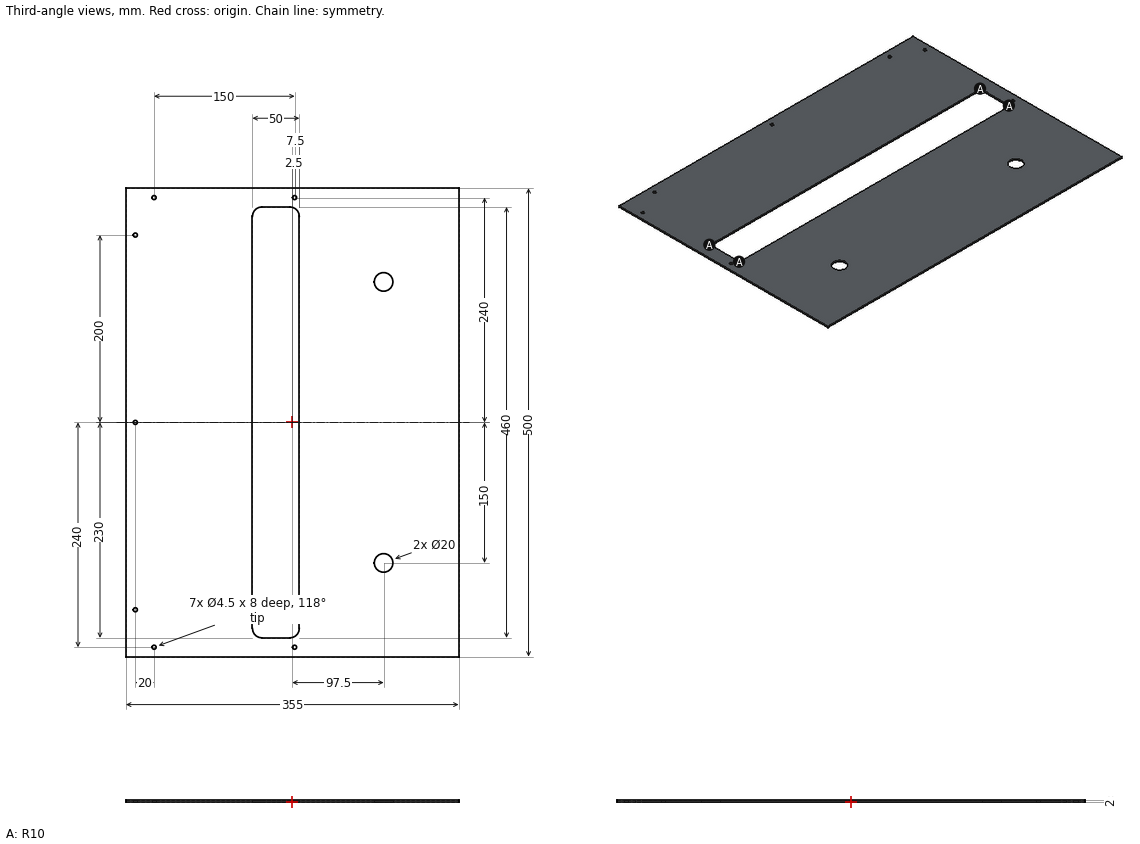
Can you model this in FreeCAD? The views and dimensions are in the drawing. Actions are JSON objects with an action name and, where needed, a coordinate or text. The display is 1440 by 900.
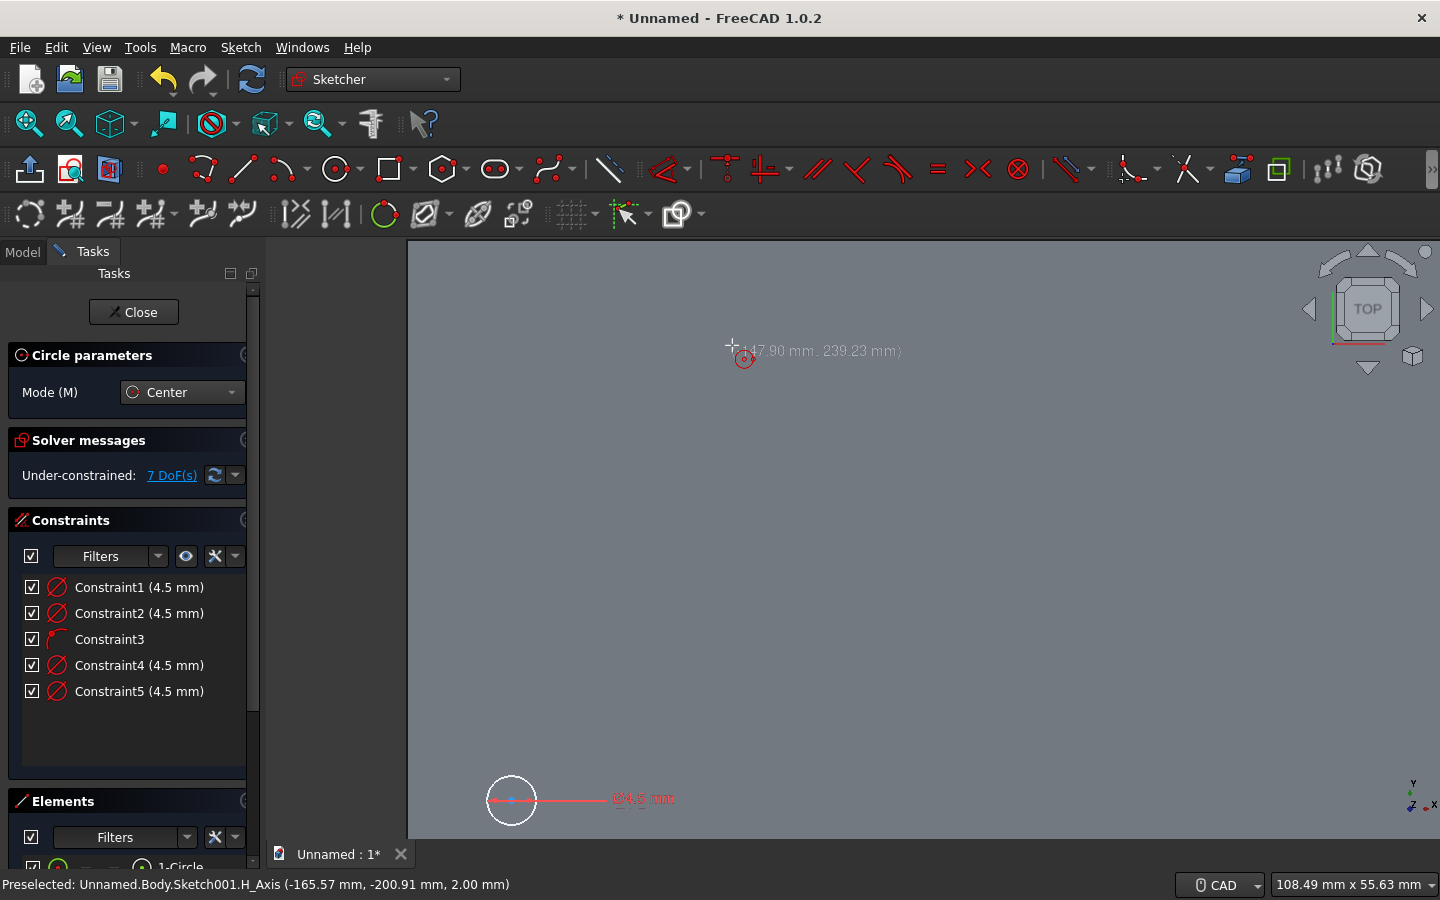
{"action": "scroll", "coordinate": [732, 345], "scroll_direction": "down", "scroll_amount": 13}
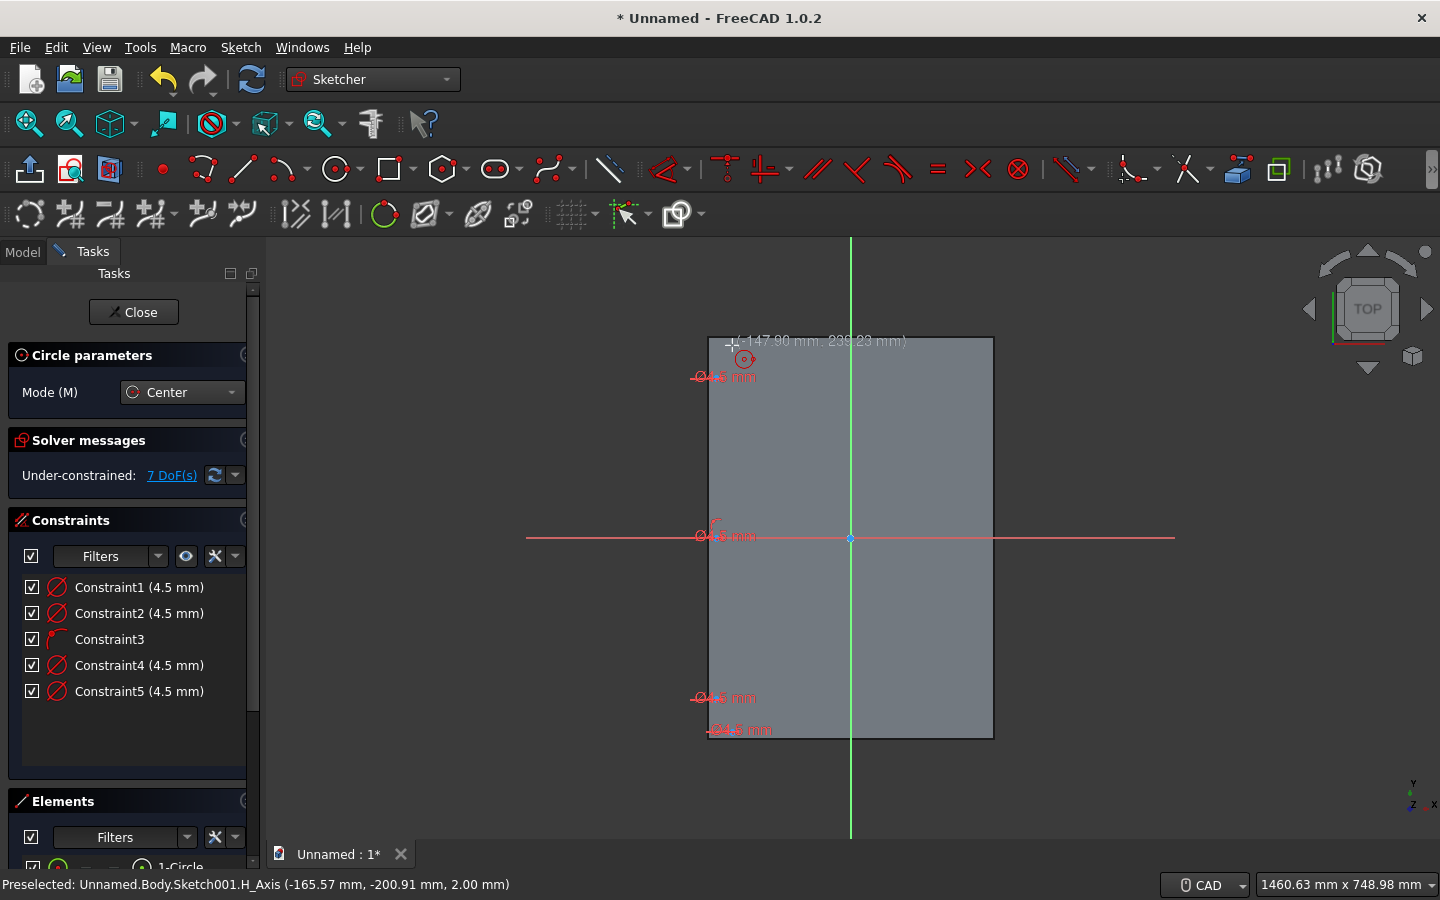
{"action": "left_click", "coordinate": [732, 345]}
{"action": "mouse_move", "coordinate": [734, 344]}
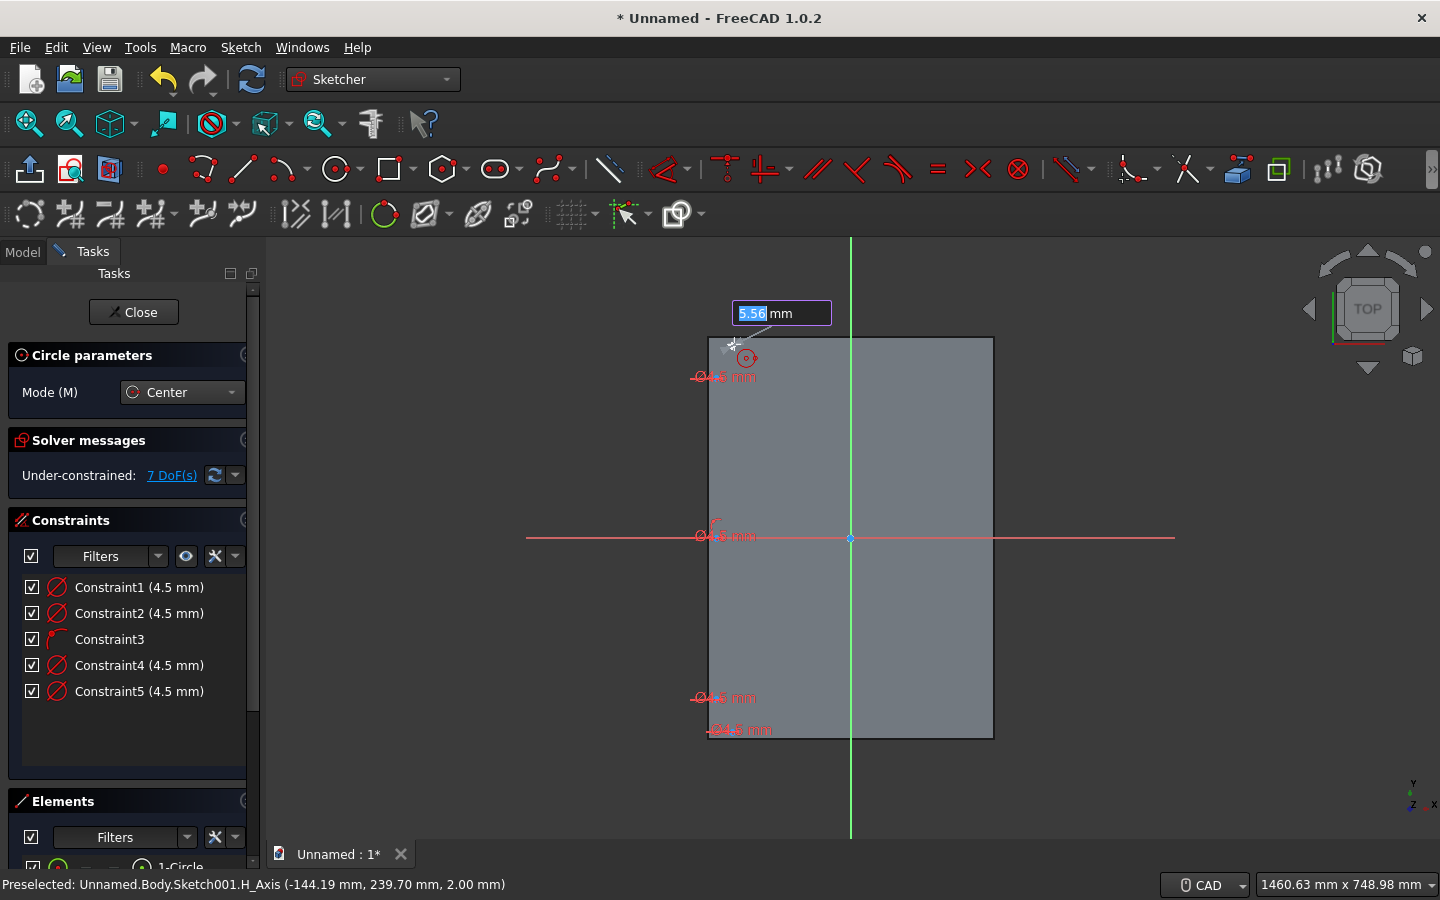
{"action": "type", "text": "4.5"}
{"action": "key", "text": "Return"}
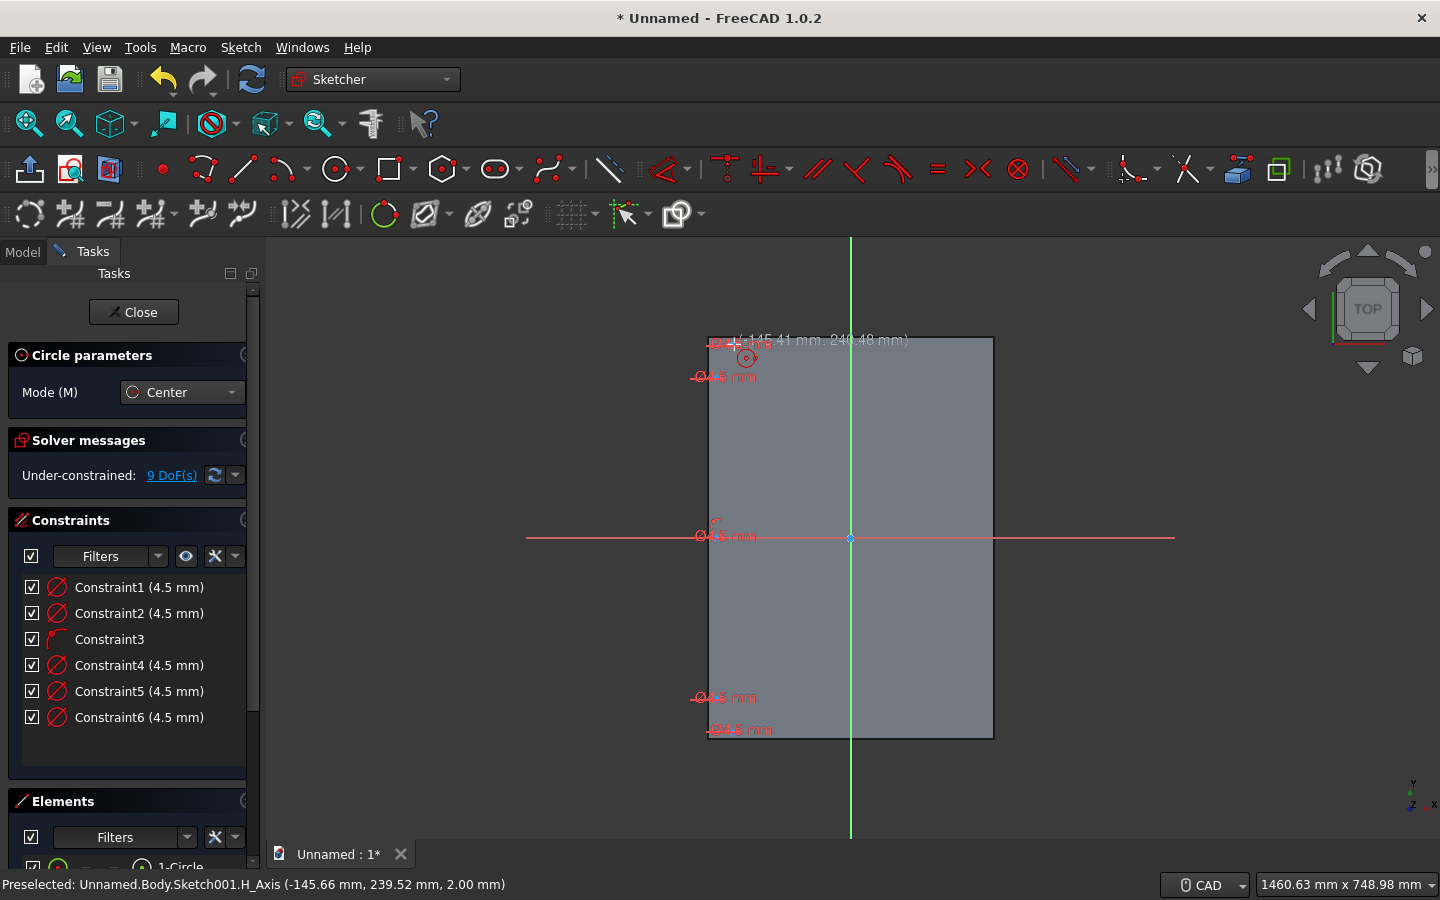
{"action": "scroll", "coordinate": [853, 345], "scroll_direction": "up", "scroll_amount": 13}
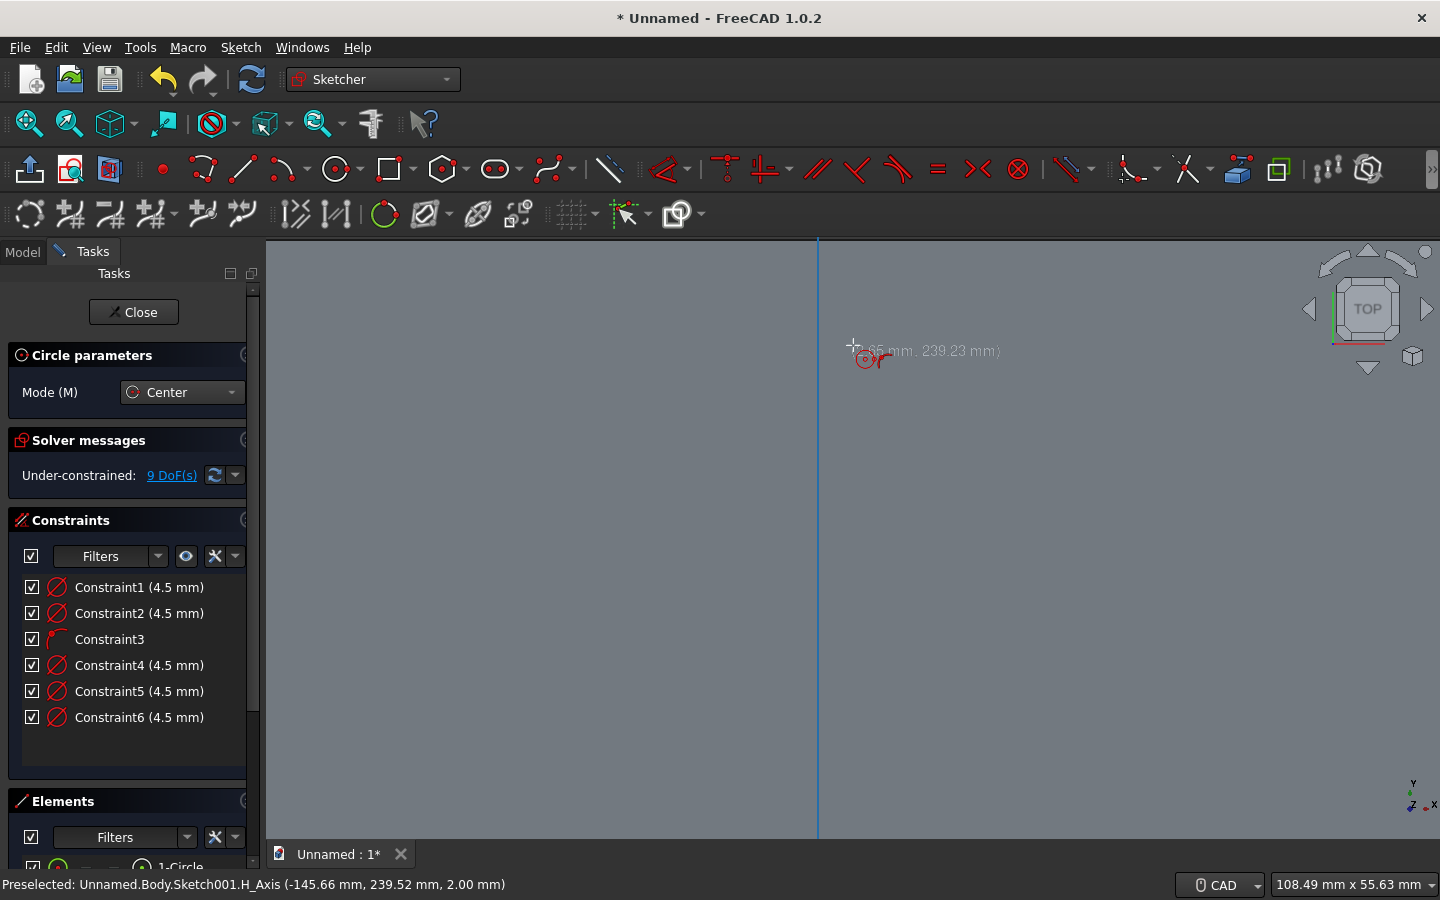
{"action": "left_click", "coordinate": [845, 348]}
{"action": "mouse_move", "coordinate": [862, 331]}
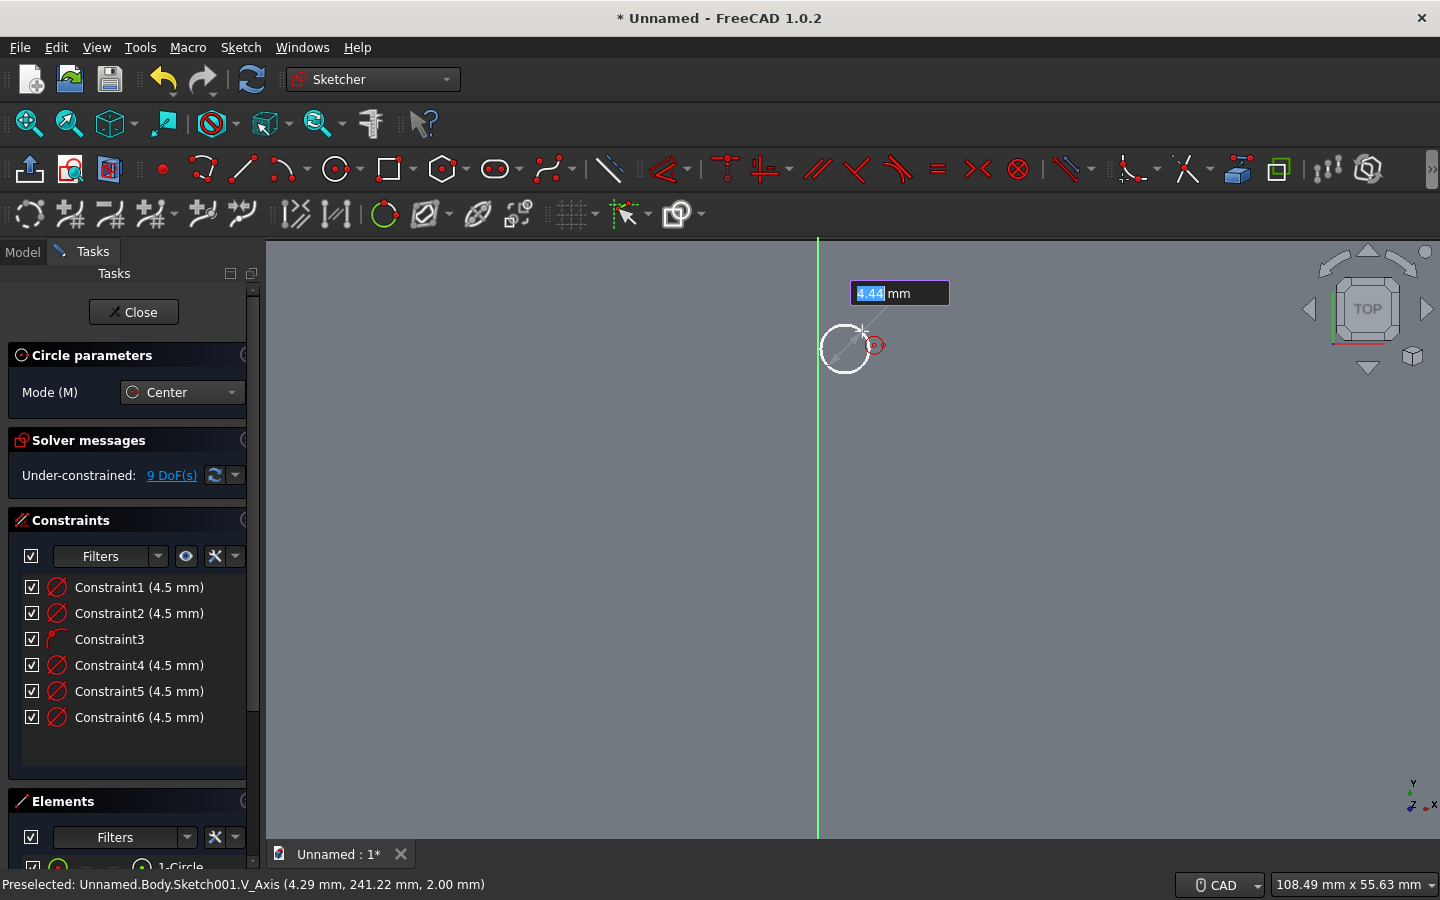
{"action": "type", "text": "4.5"}
{"action": "key", "text": "Return"}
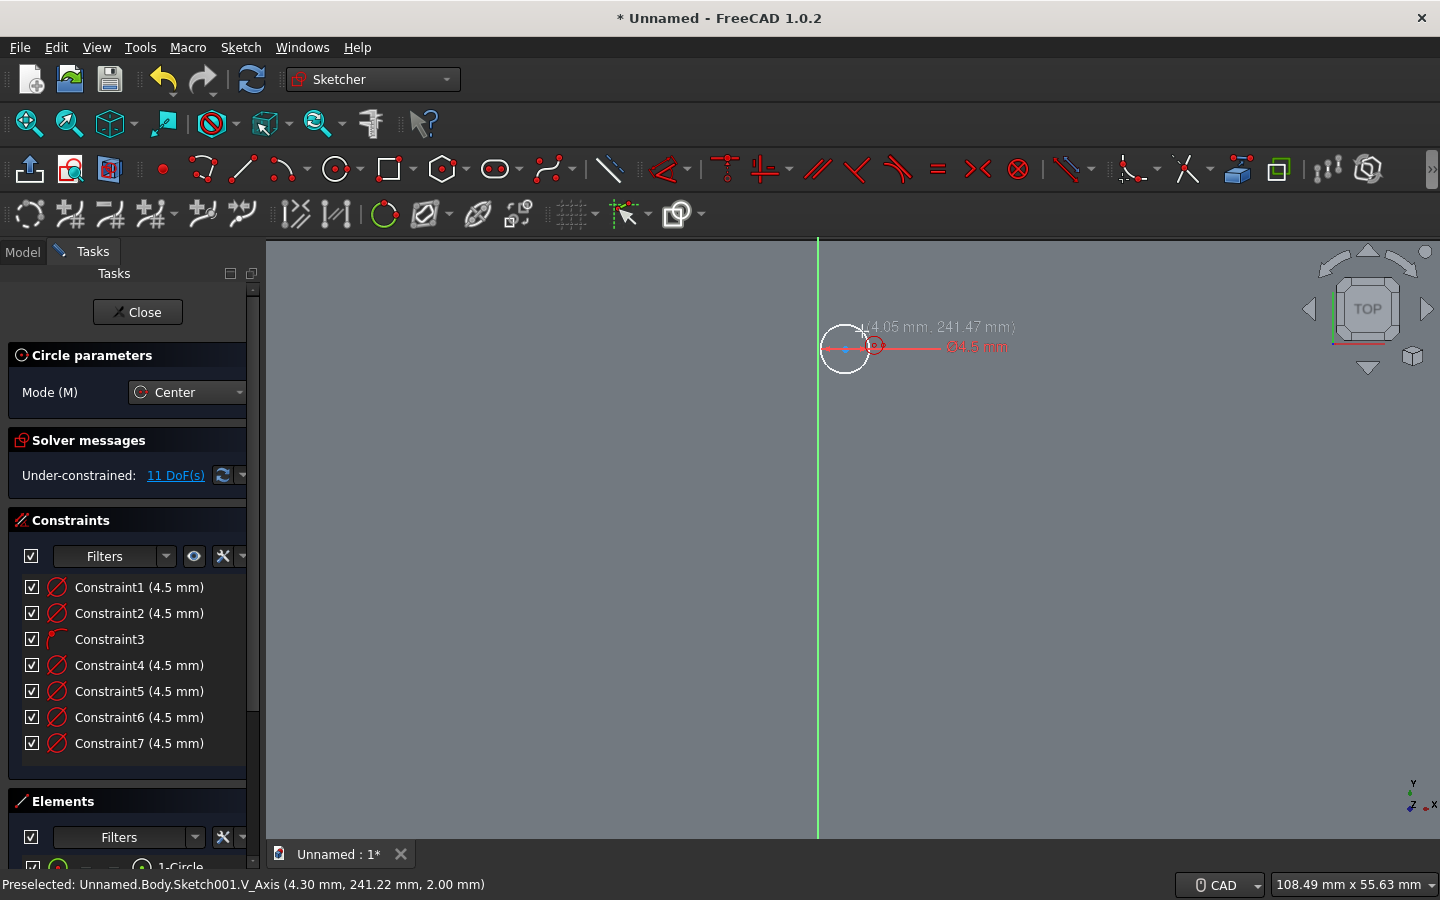
{"action": "scroll", "coordinate": [853, 345], "scroll_direction": "down", "scroll_amount": 13}